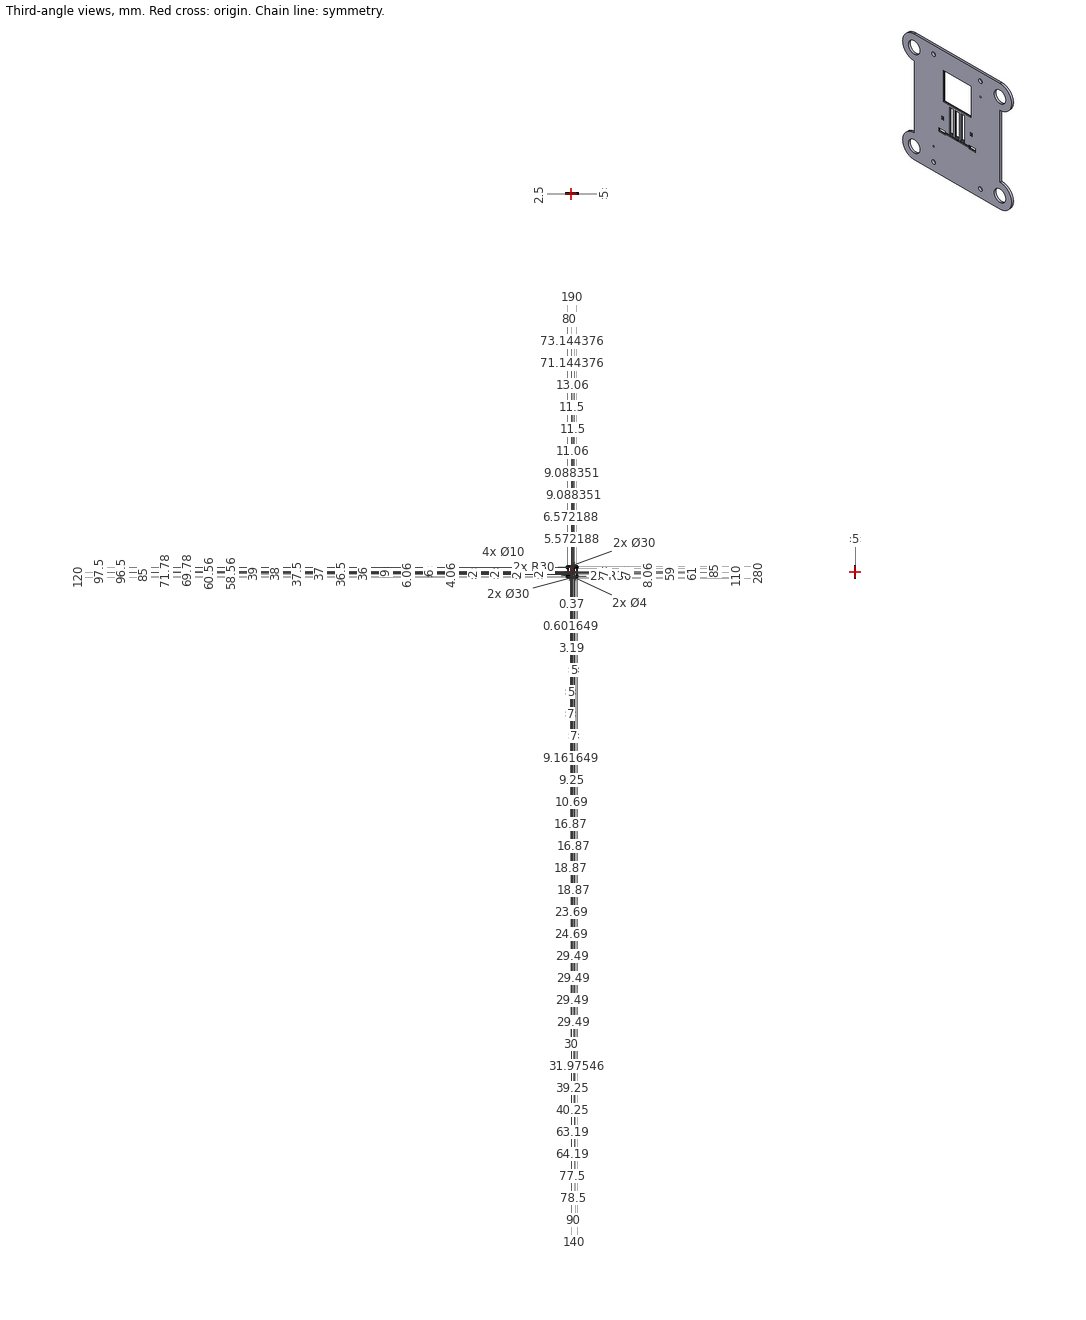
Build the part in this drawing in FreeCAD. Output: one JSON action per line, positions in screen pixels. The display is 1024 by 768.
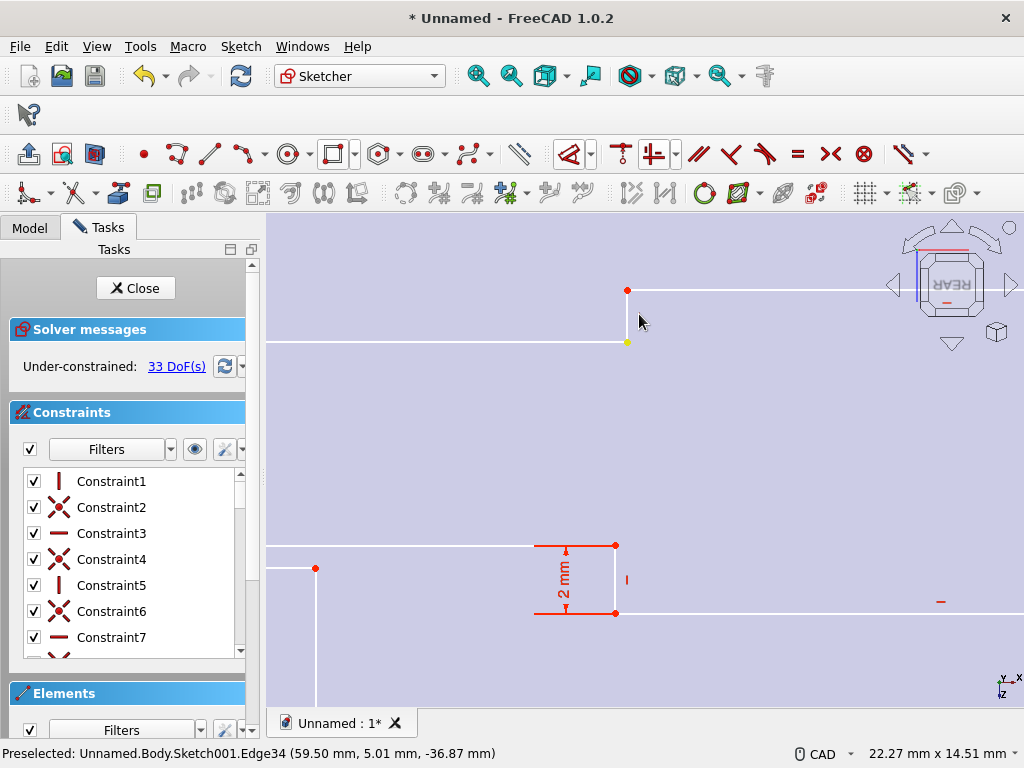
{"action": "left_click", "coordinate": [627, 306]}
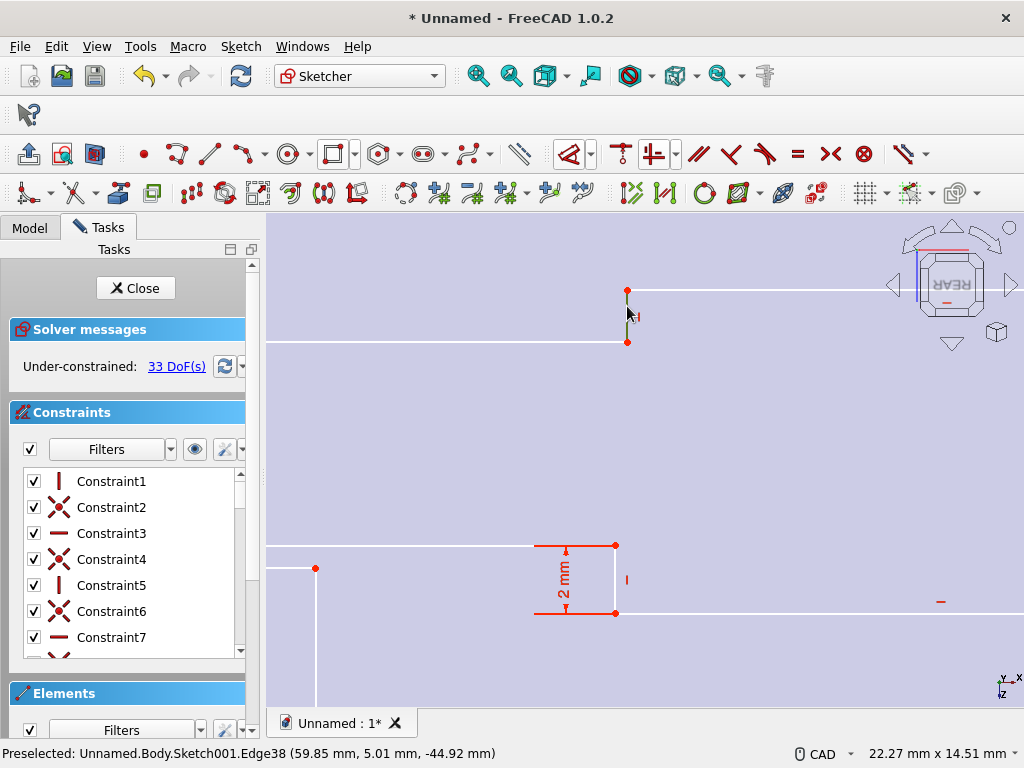
{"action": "key", "text": "i"}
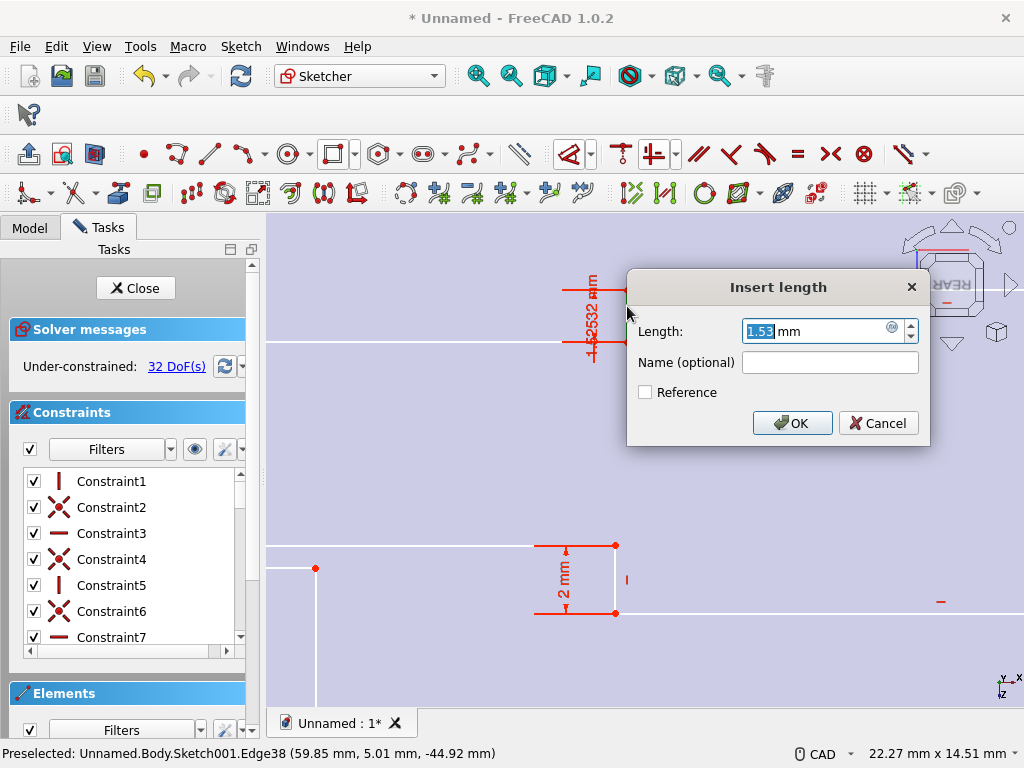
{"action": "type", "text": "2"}
{"action": "key", "text": "Return"}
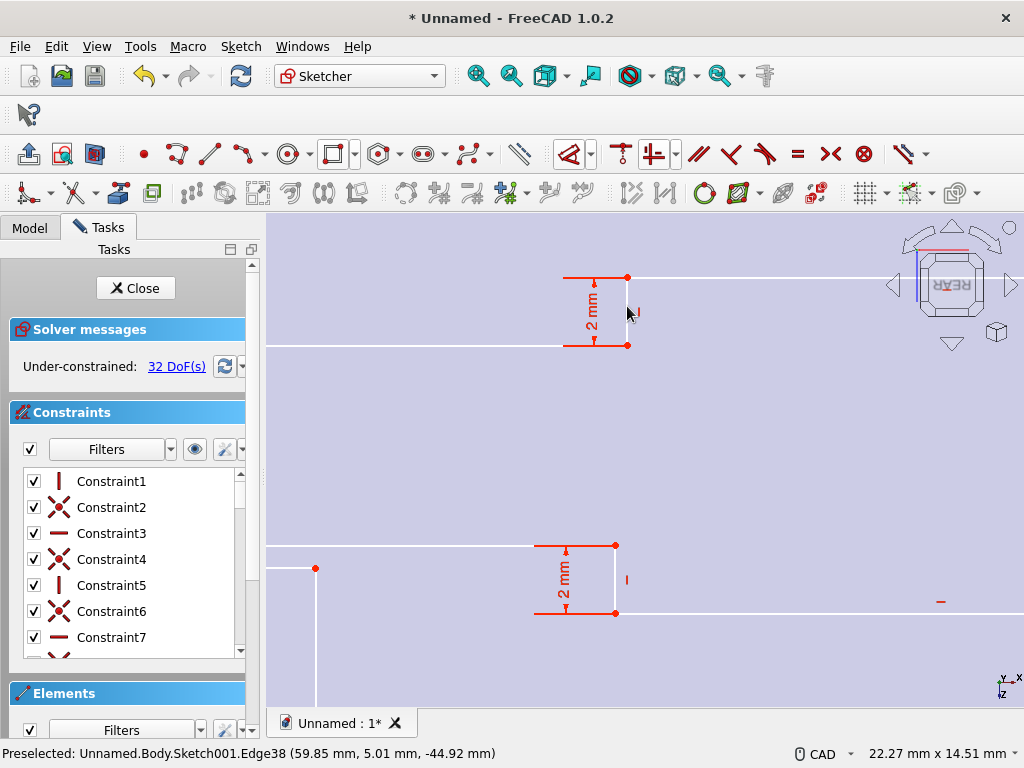
{"action": "scroll", "coordinate": [639, 314], "scroll_direction": "down", "scroll_amount": 14}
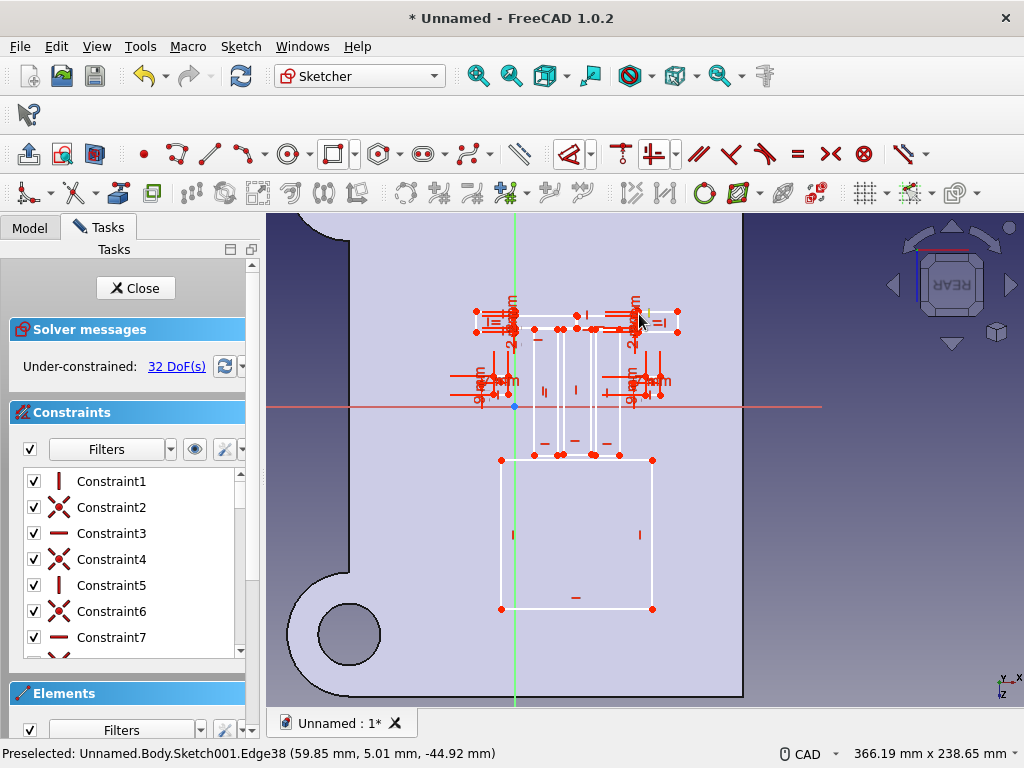
{"action": "scroll", "coordinate": [596, 367], "scroll_direction": "up", "scroll_amount": 6}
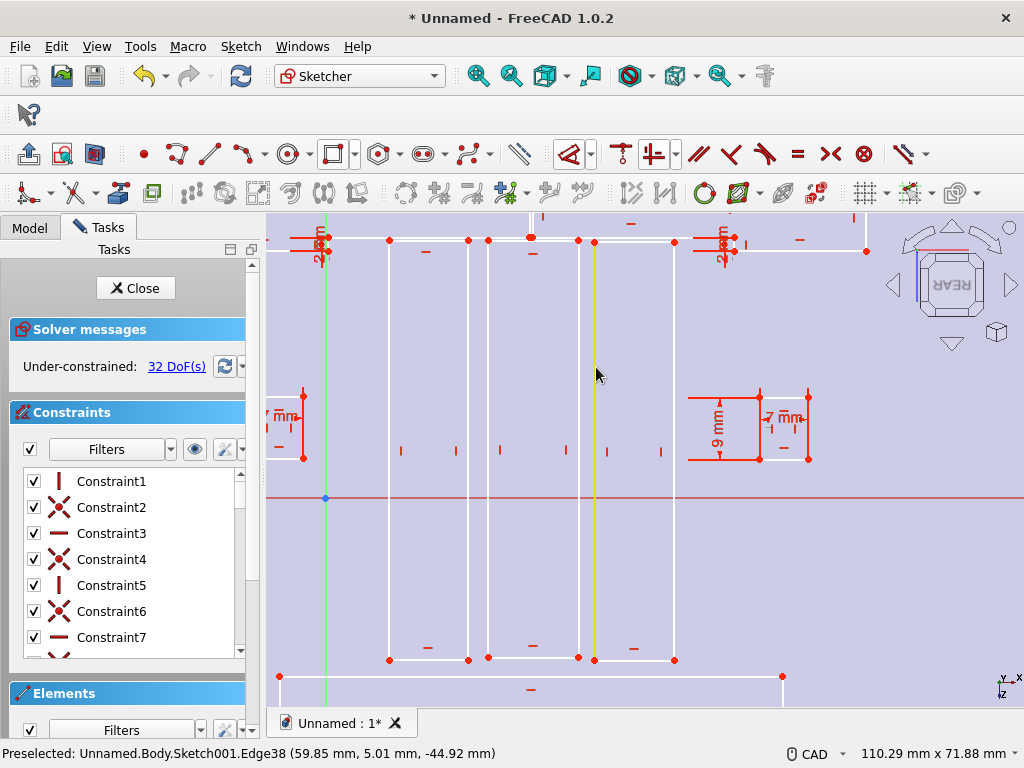
{"action": "left_click", "coordinate": [595, 368]}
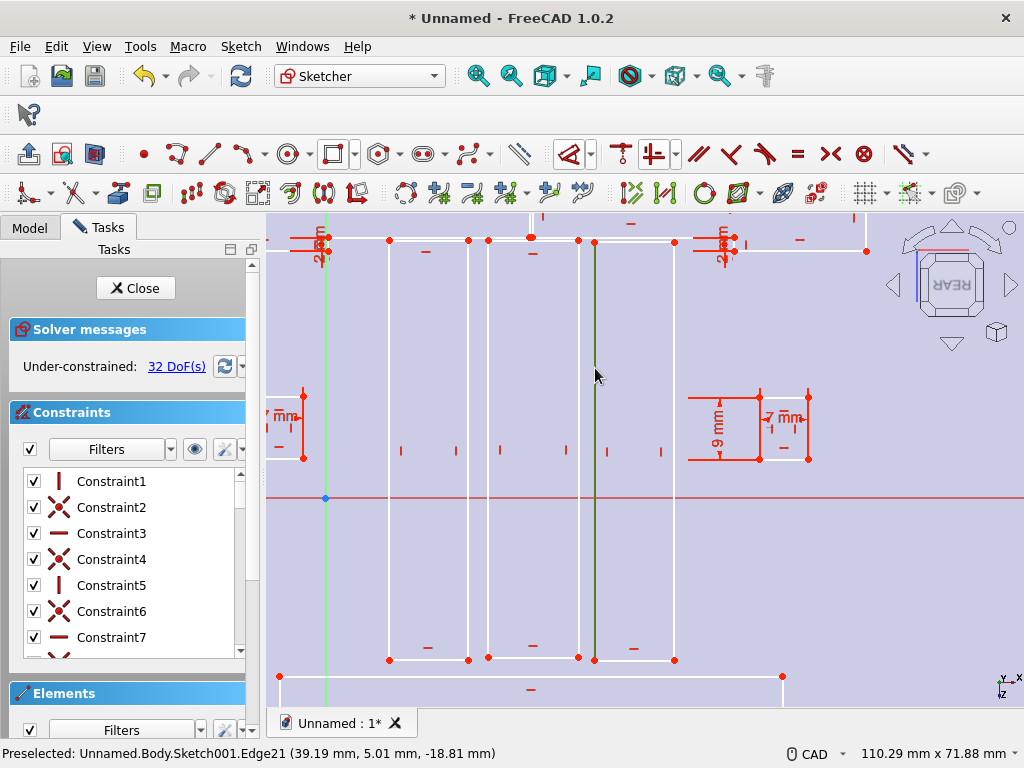
{"action": "left_click", "coordinate": [590, 154]}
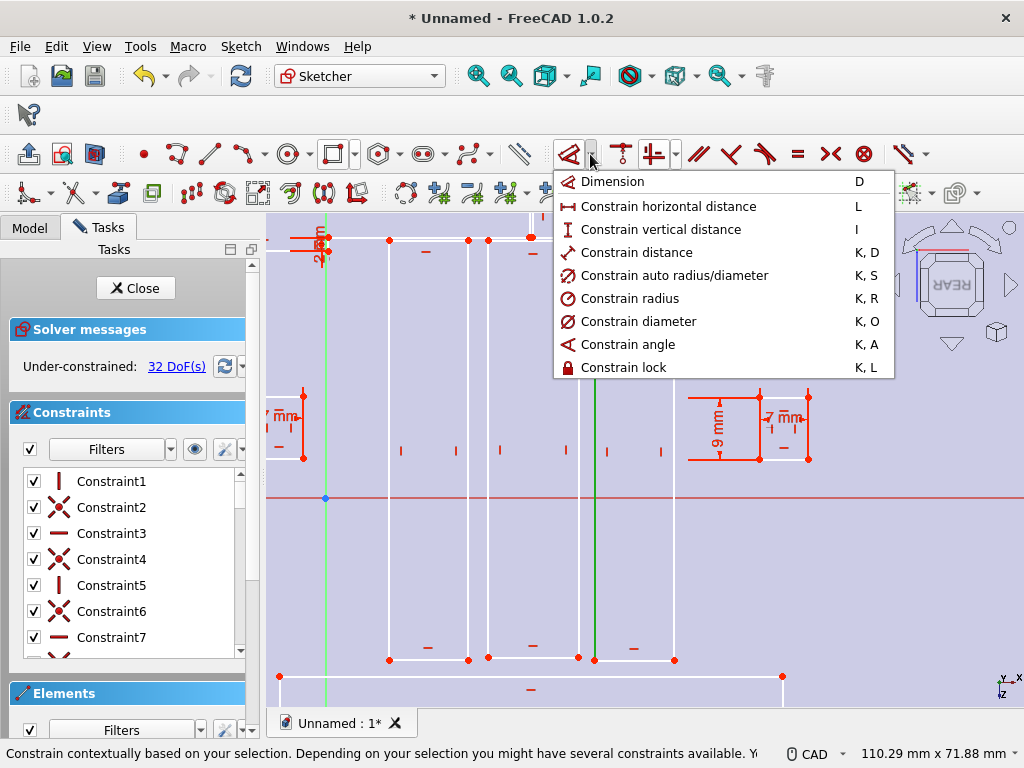
{"action": "left_click", "coordinate": [724, 230]}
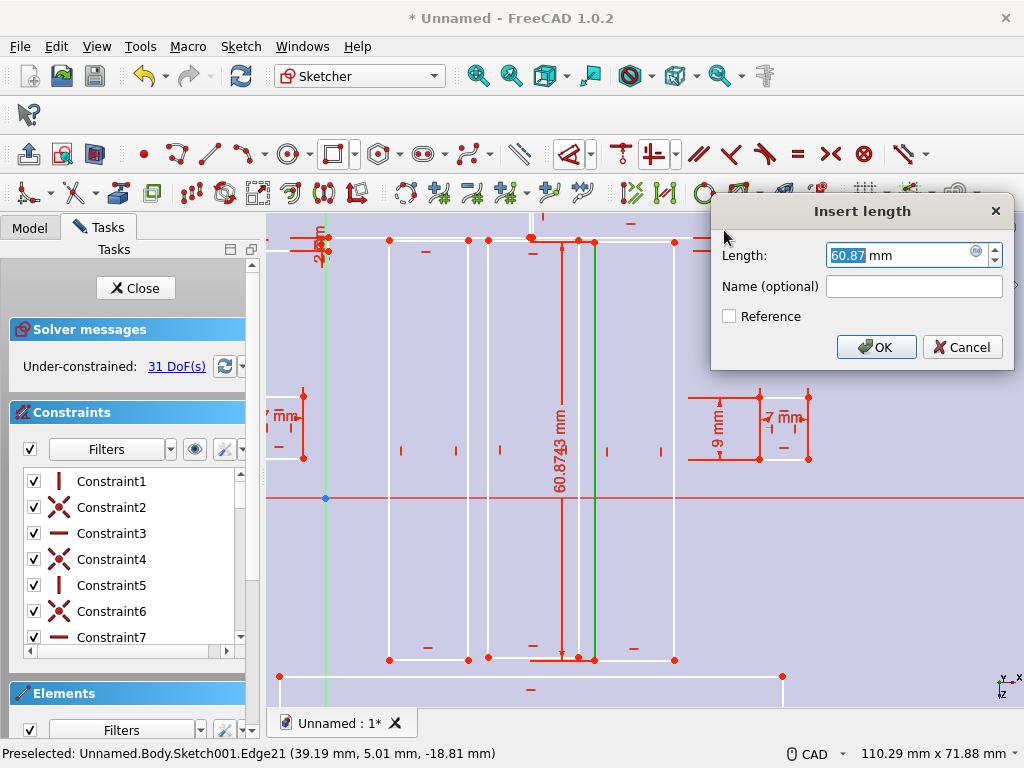
{"action": "type", "text": "61"}
{"action": "key", "text": "Return"}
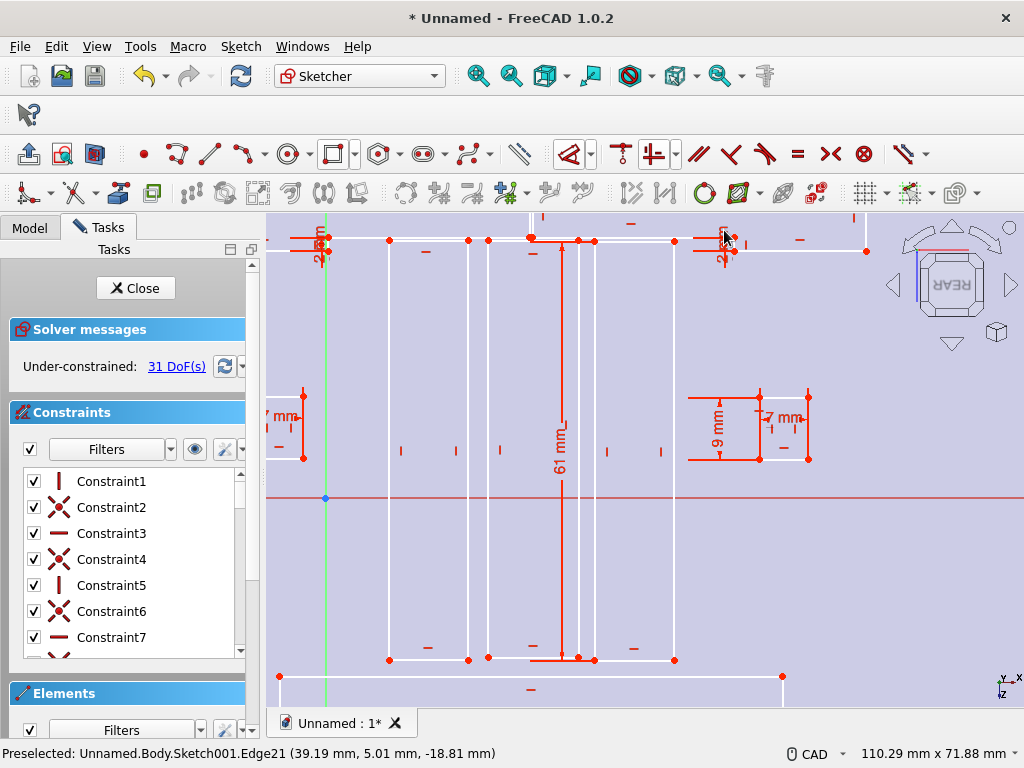
{"action": "left_click", "coordinate": [389, 367]}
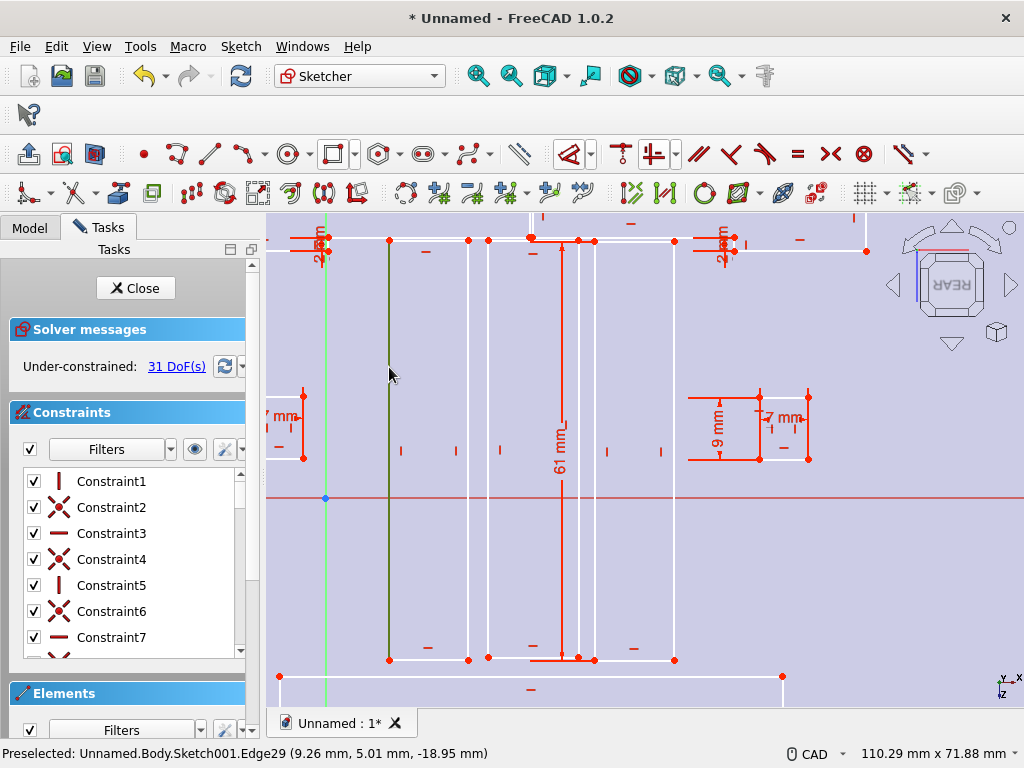
{"action": "key", "text": "i"}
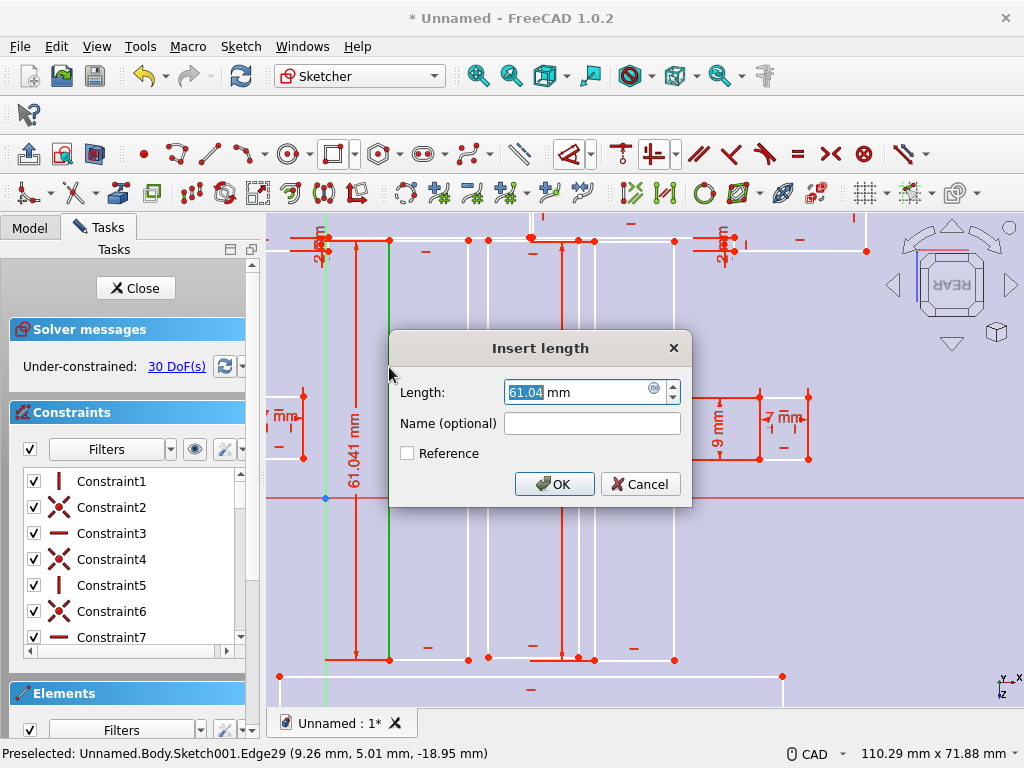
{"action": "type", "text": "61"}
{"action": "key", "text": "Return"}